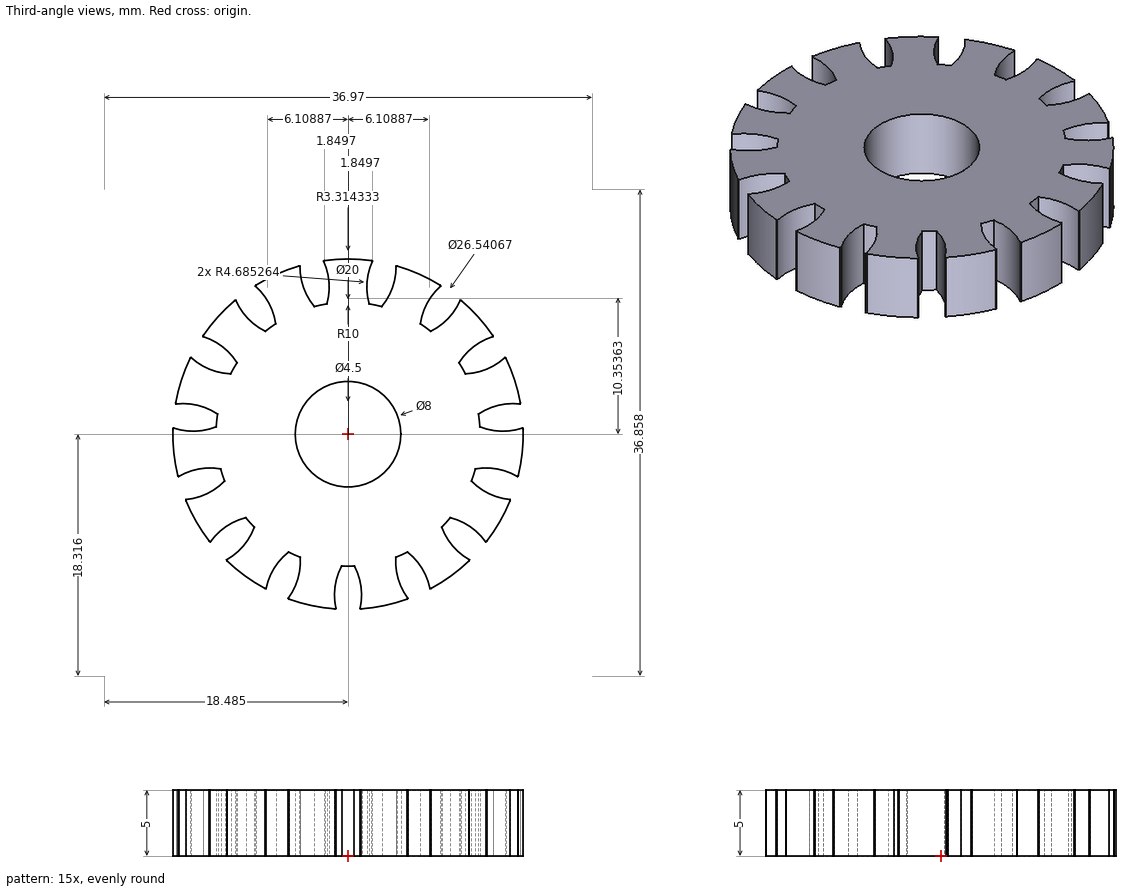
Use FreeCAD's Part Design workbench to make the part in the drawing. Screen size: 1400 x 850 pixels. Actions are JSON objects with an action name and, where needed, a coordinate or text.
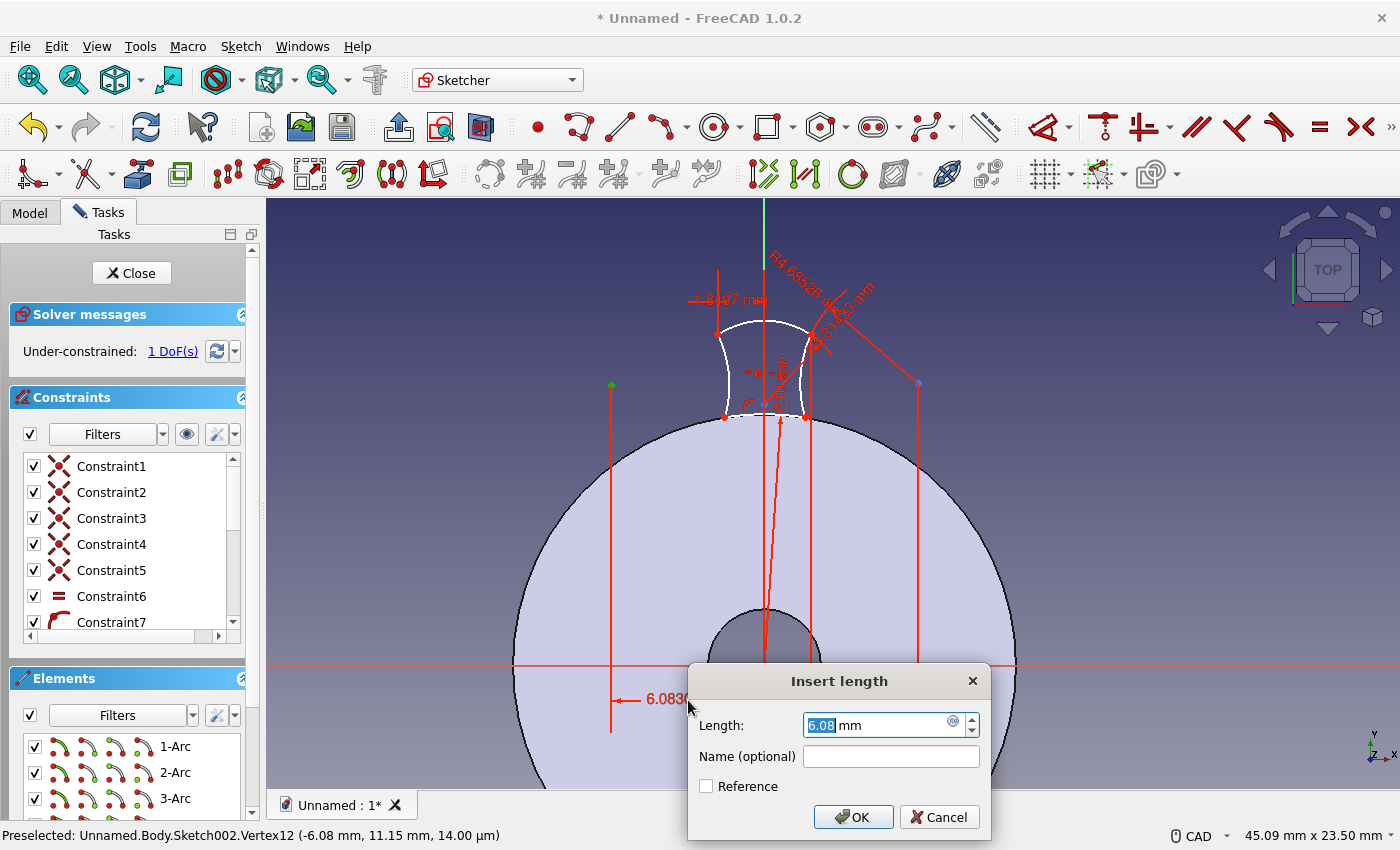
{"action": "type", "text": "6.10887"}
{"action": "key", "text": "Return"}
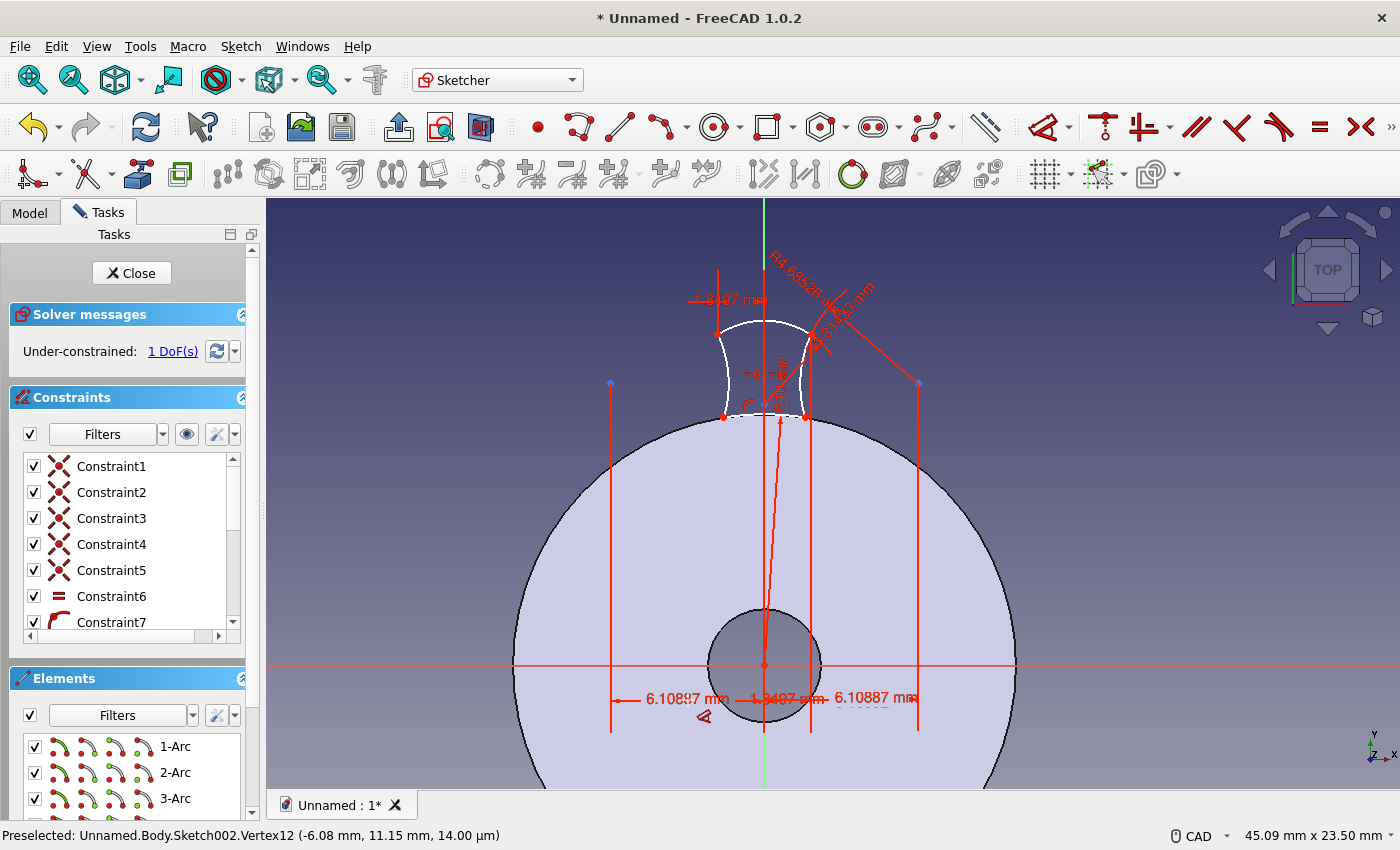
{"action": "left_click", "coordinate": [764, 404]}
{"action": "left_click", "coordinate": [798, 535]}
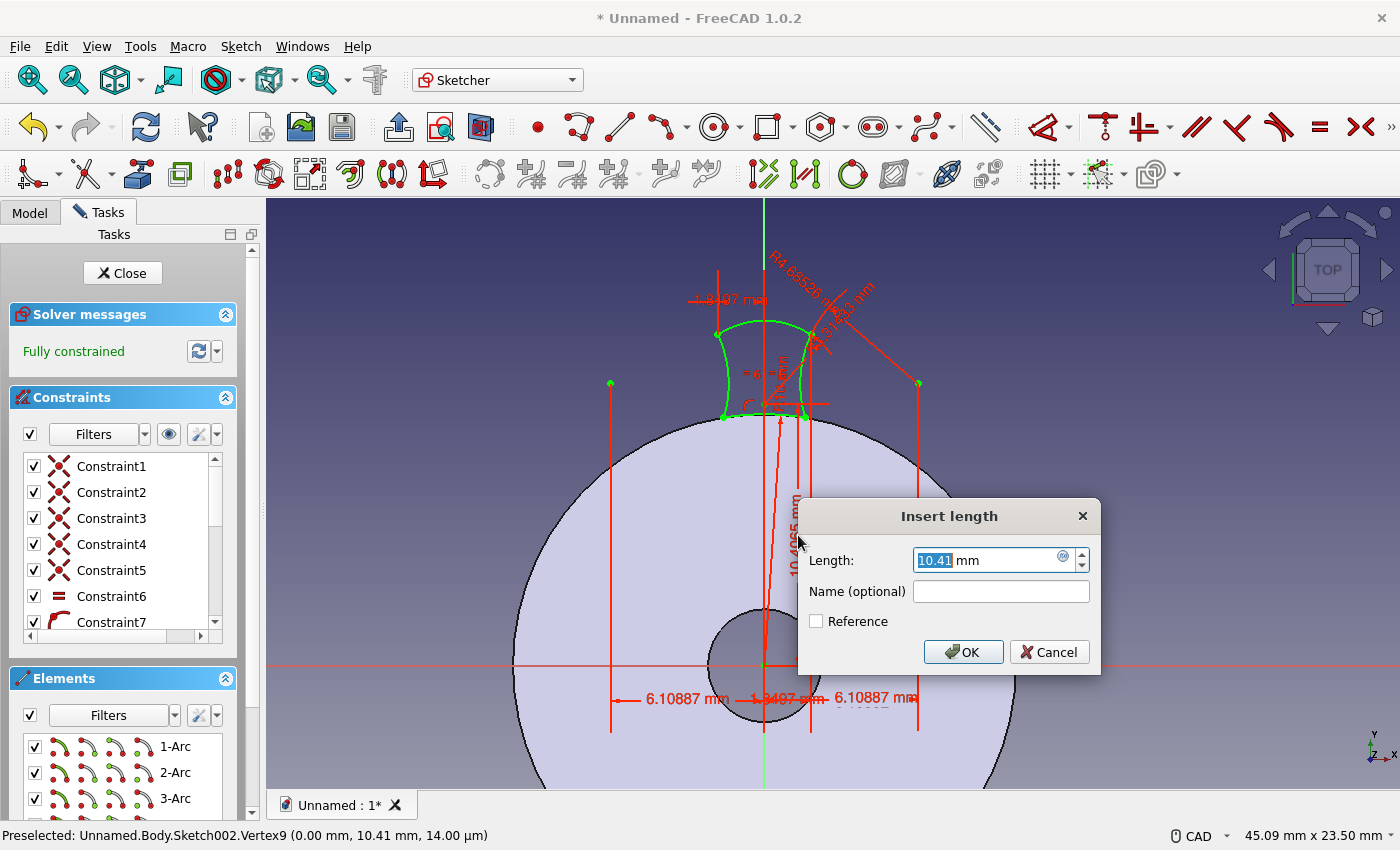
{"action": "type", "text": "10.35363"}
{"action": "key", "text": "Return"}
{"action": "key", "text": "Escape"}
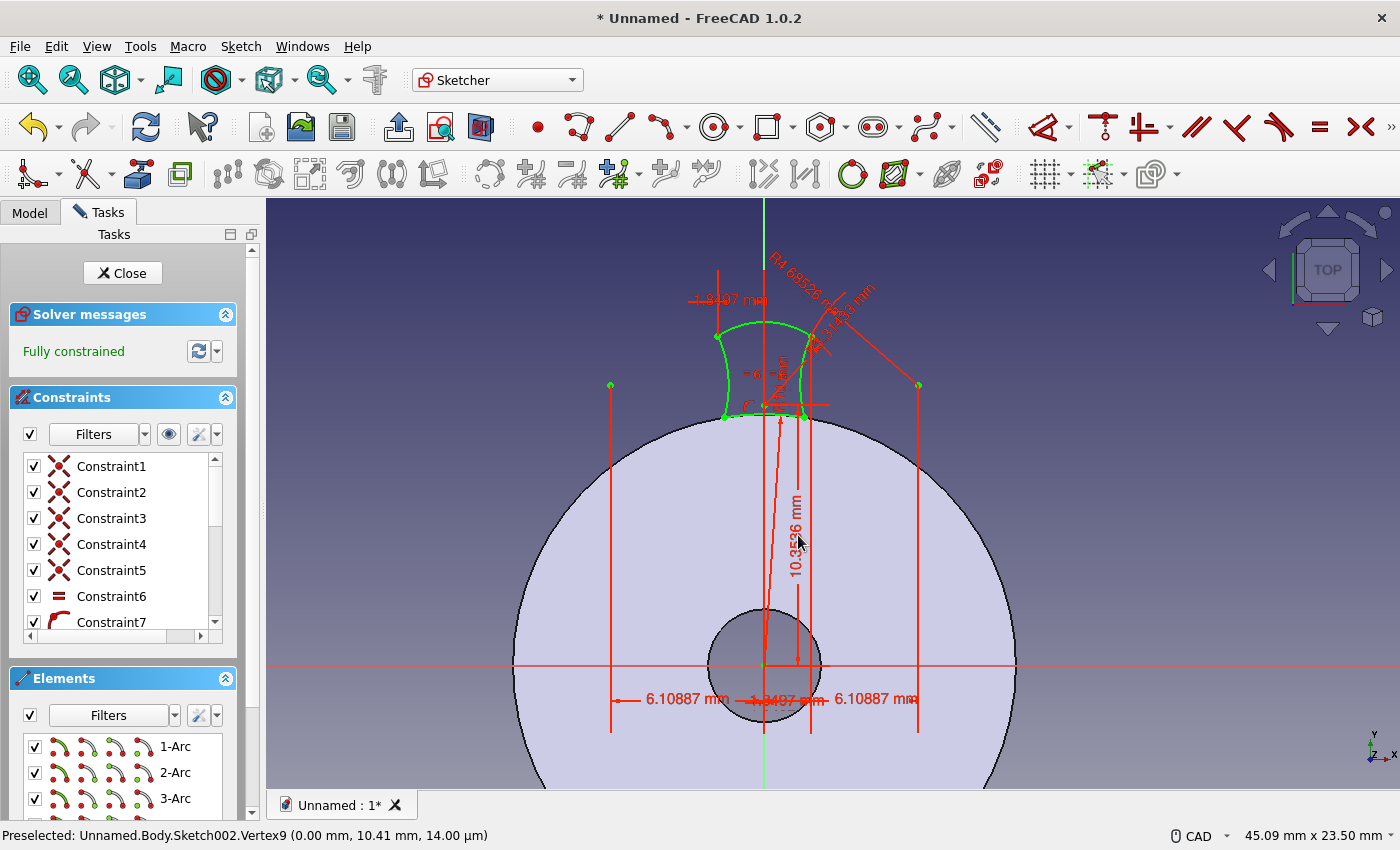
{"action": "left_click", "coordinate": [123, 273]}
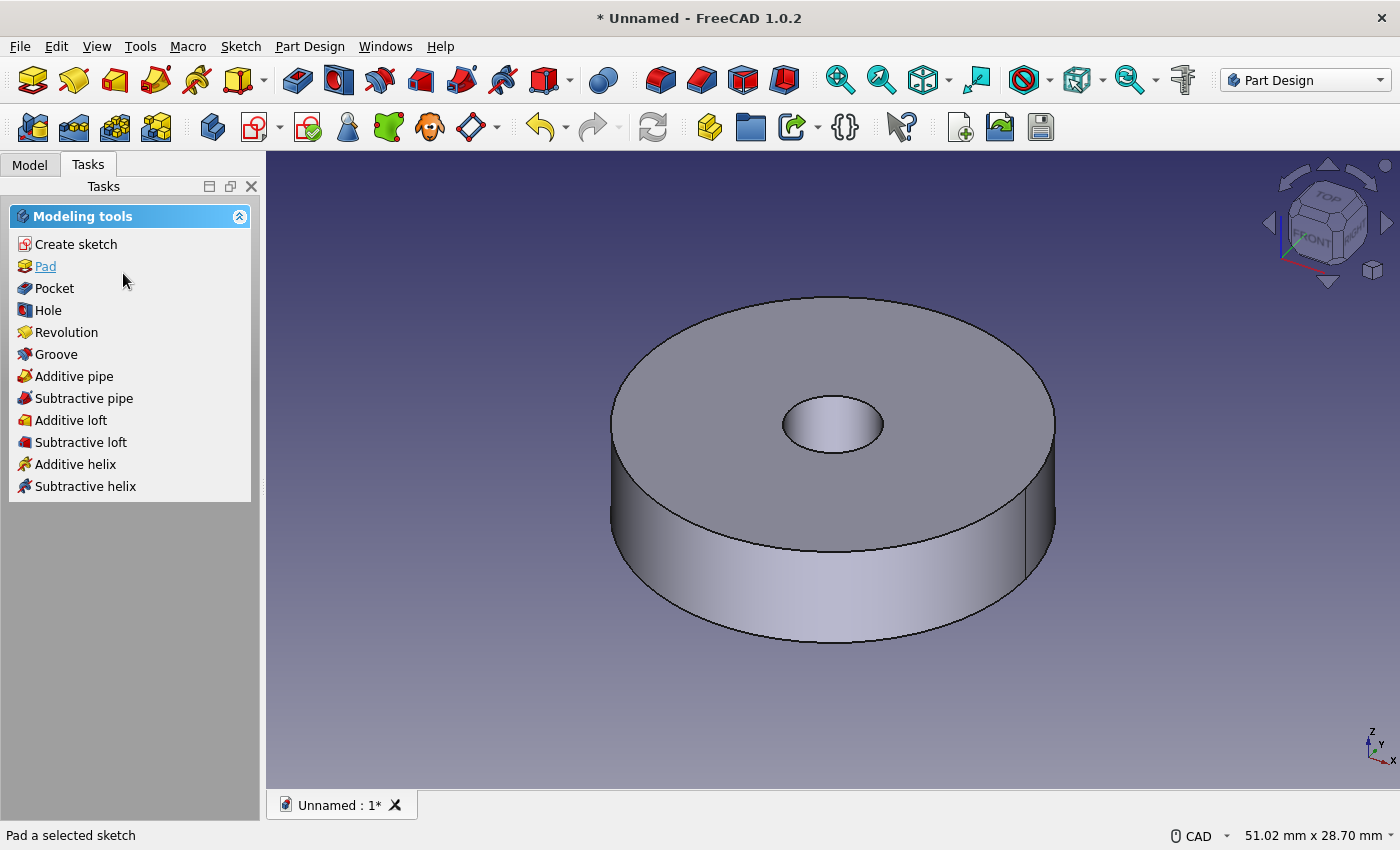
{"action": "left_click", "coordinate": [33, 80]}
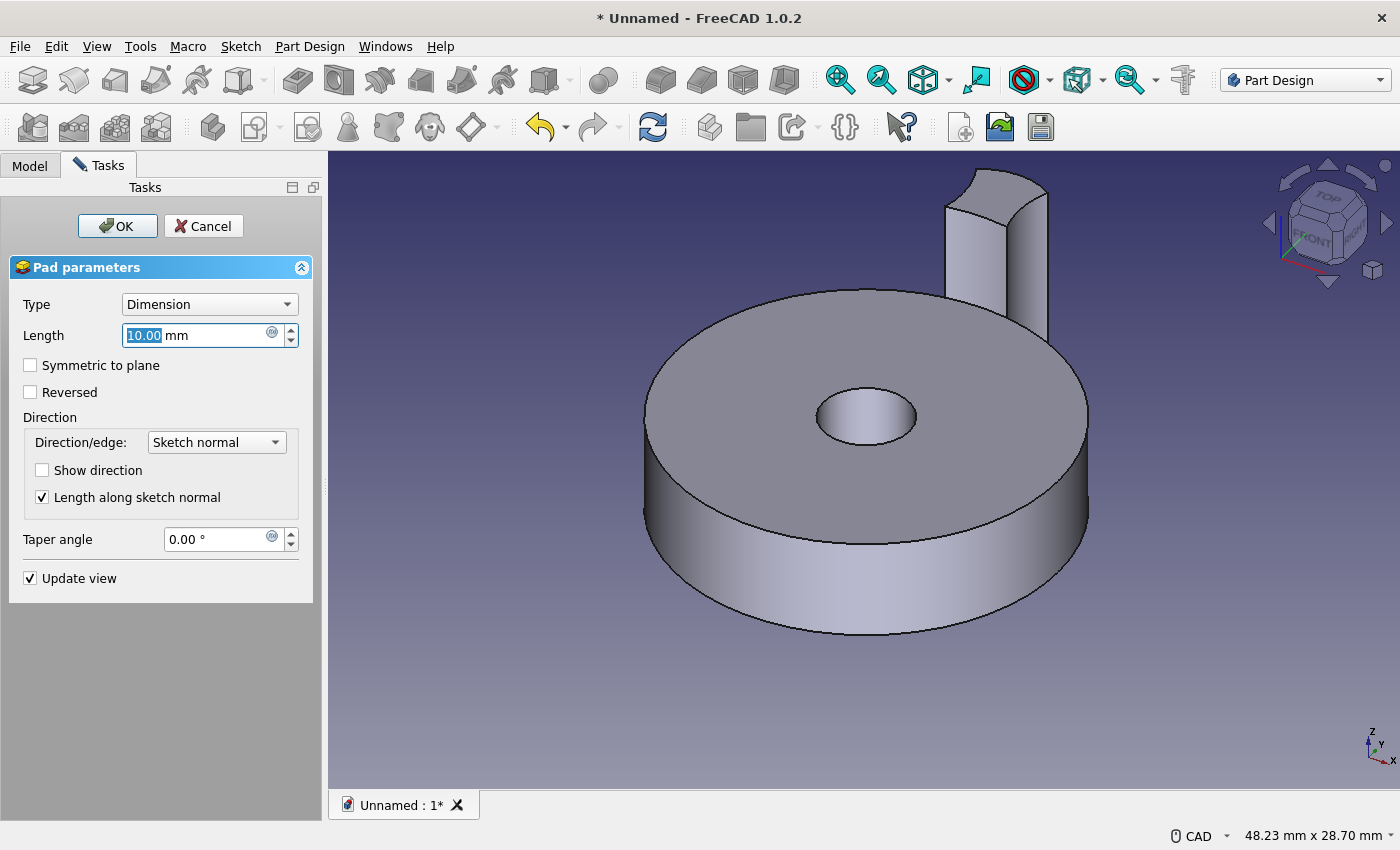
{"action": "type", "text": "5"}
{"action": "key", "text": "Tab"}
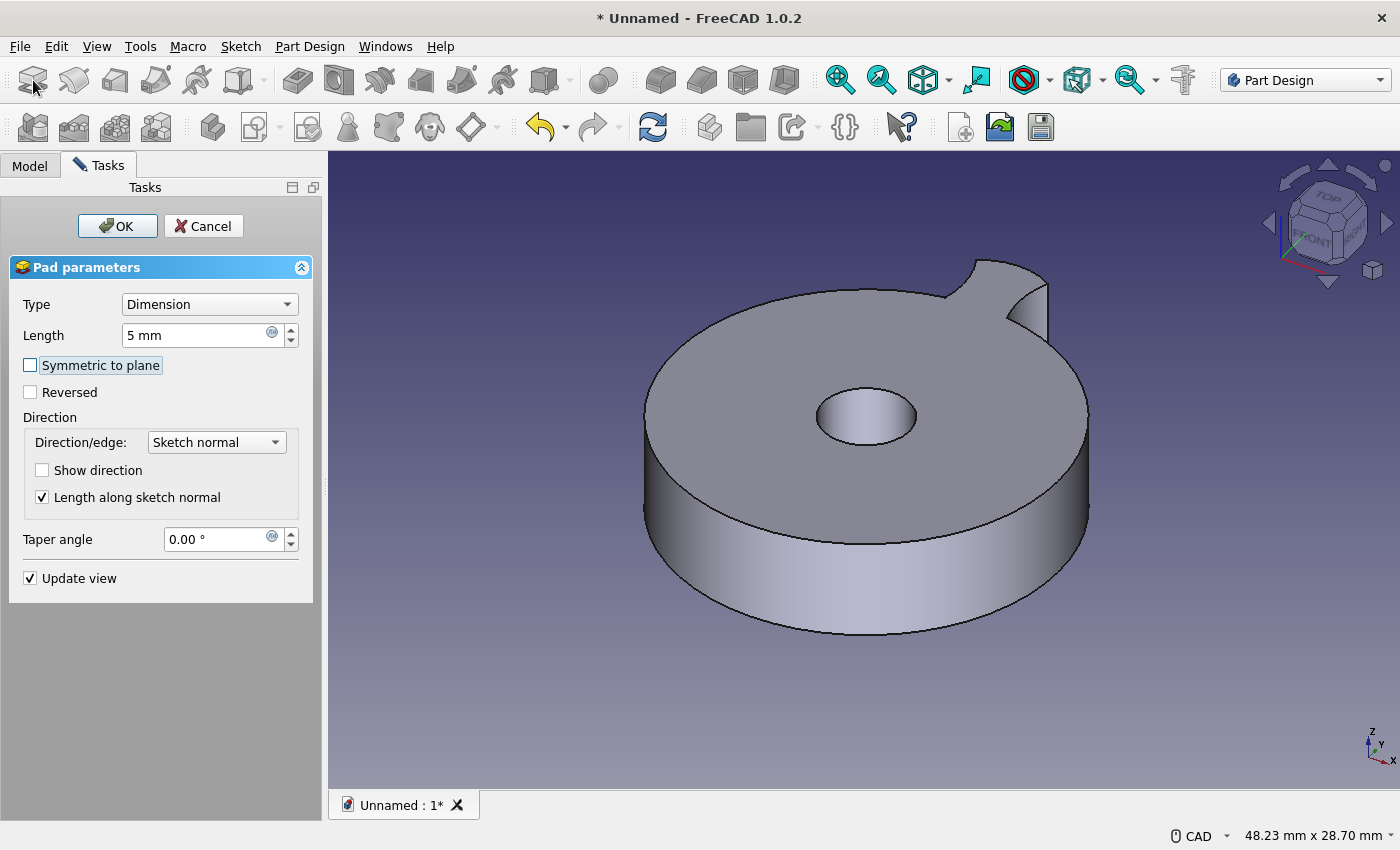
{"action": "left_click", "coordinate": [118, 226]}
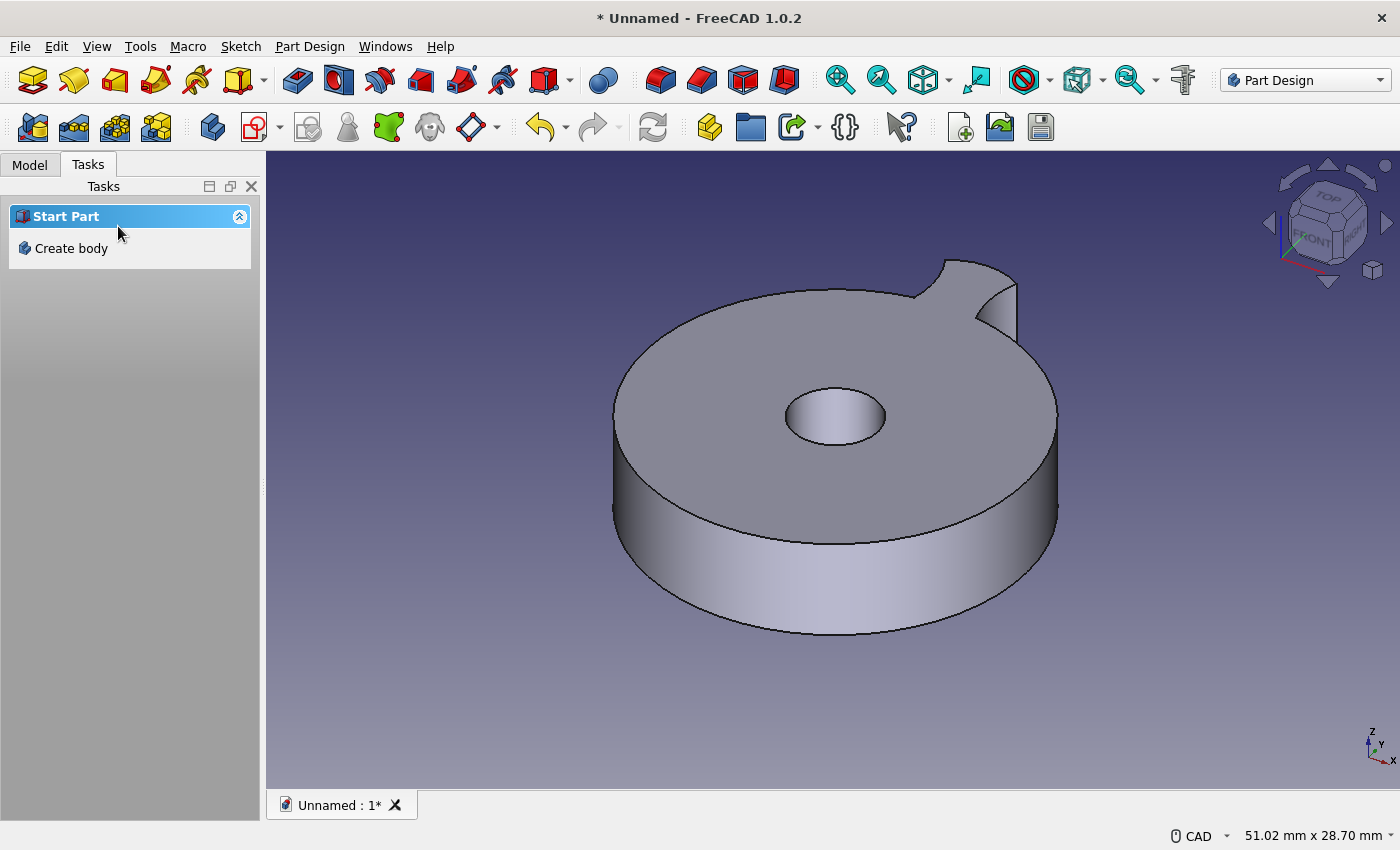
{"action": "left_click", "coordinate": [30, 164]}